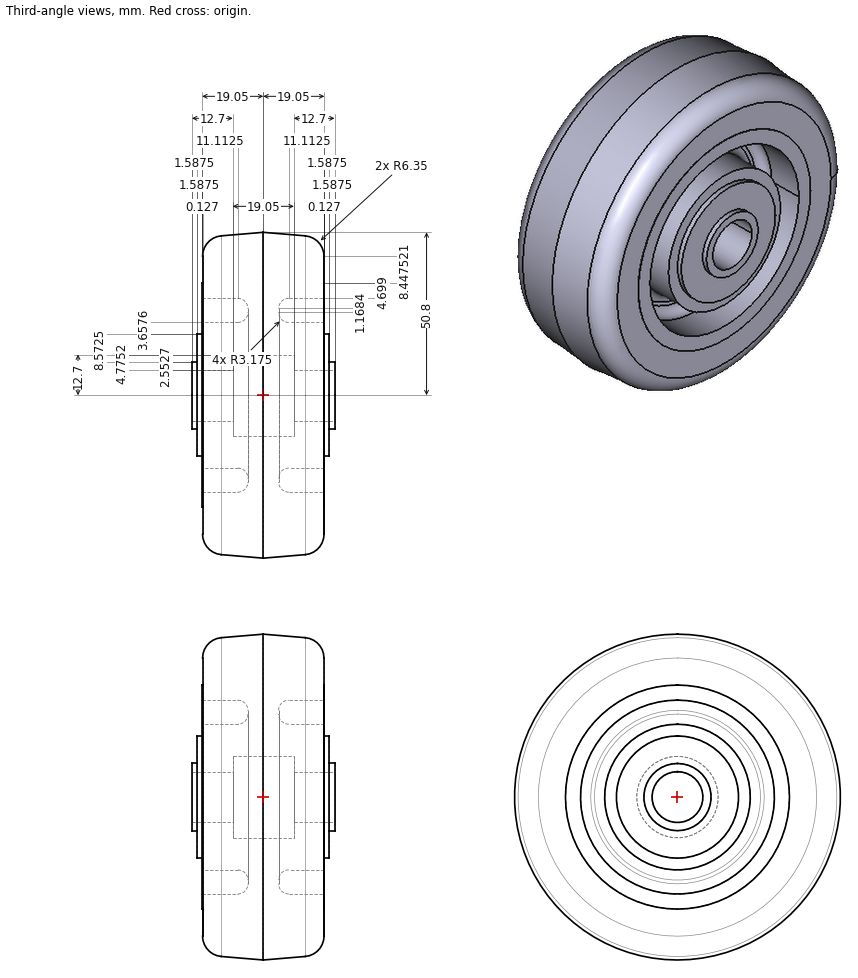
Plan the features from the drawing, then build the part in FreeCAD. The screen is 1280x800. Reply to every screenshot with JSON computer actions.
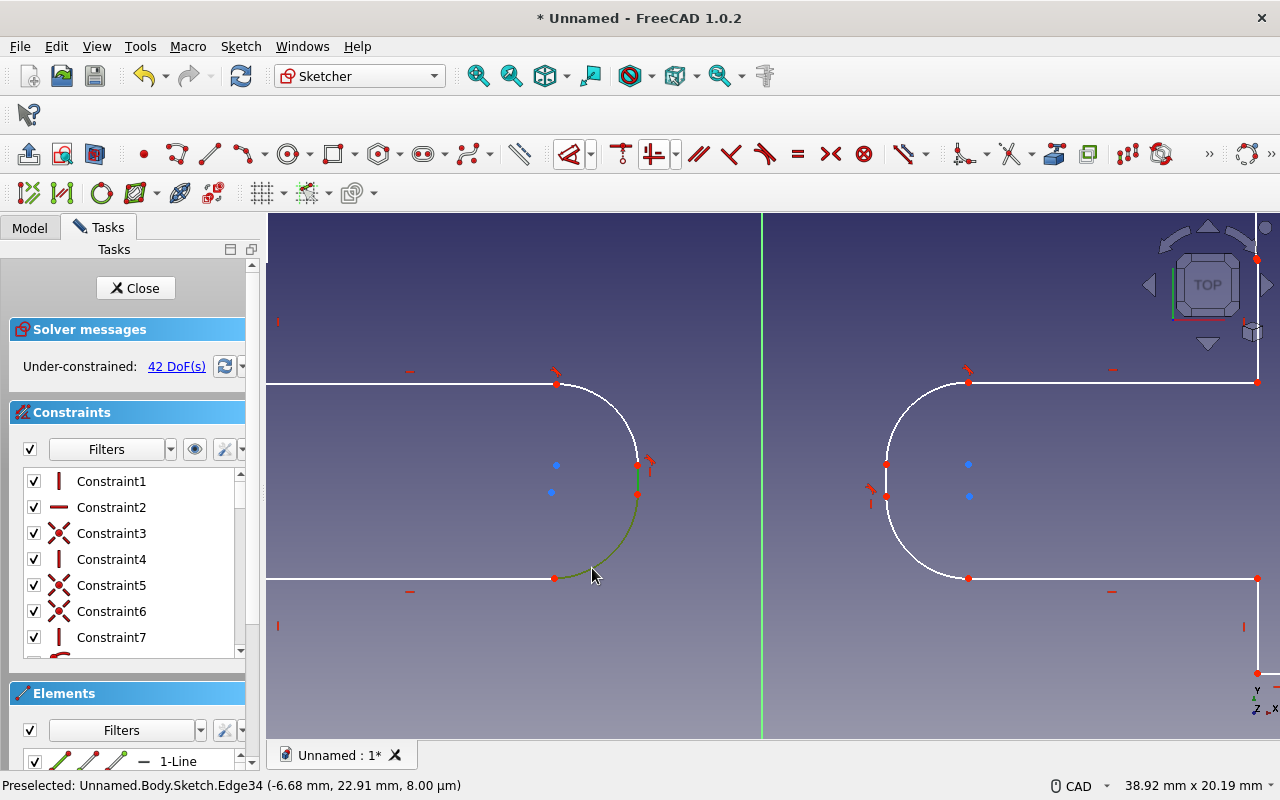
{"action": "left_click", "coordinate": [765, 154]}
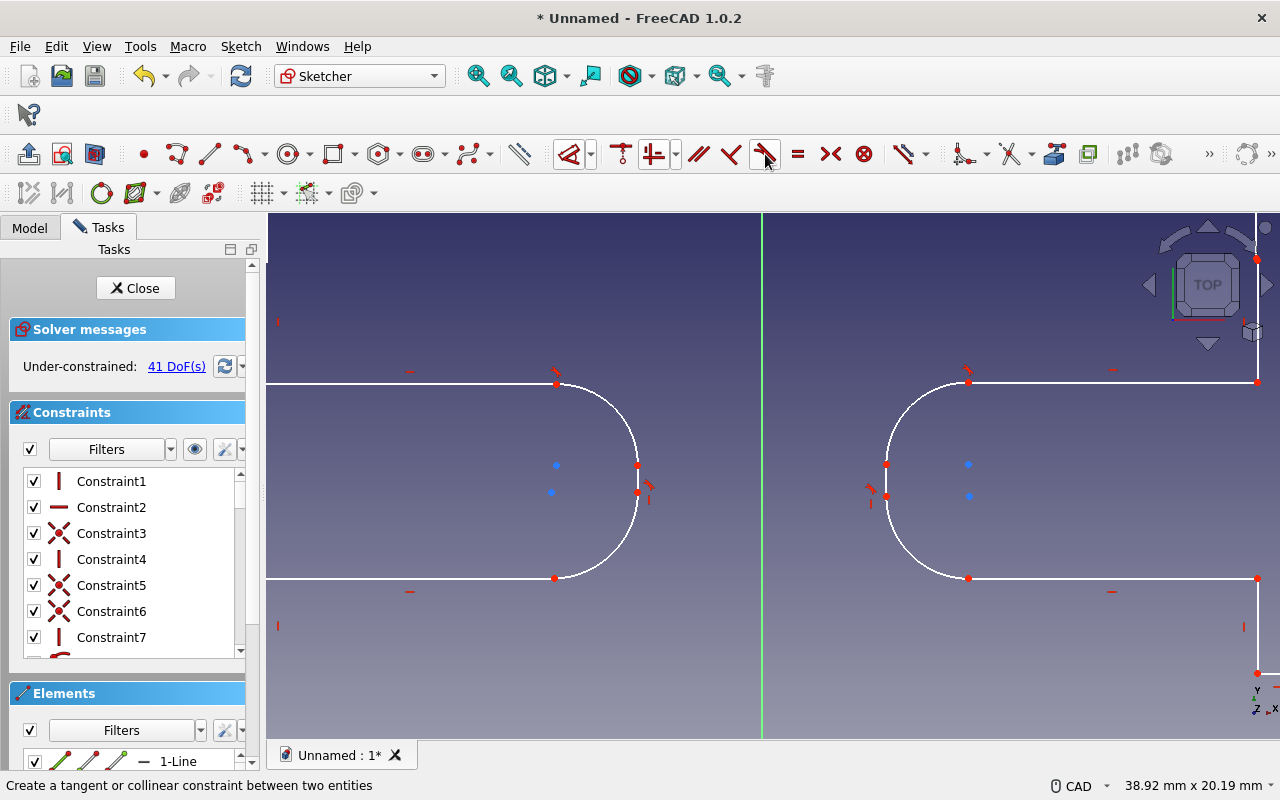
{"action": "scroll", "coordinate": [686, 466], "scroll_direction": "down", "scroll_amount": 7}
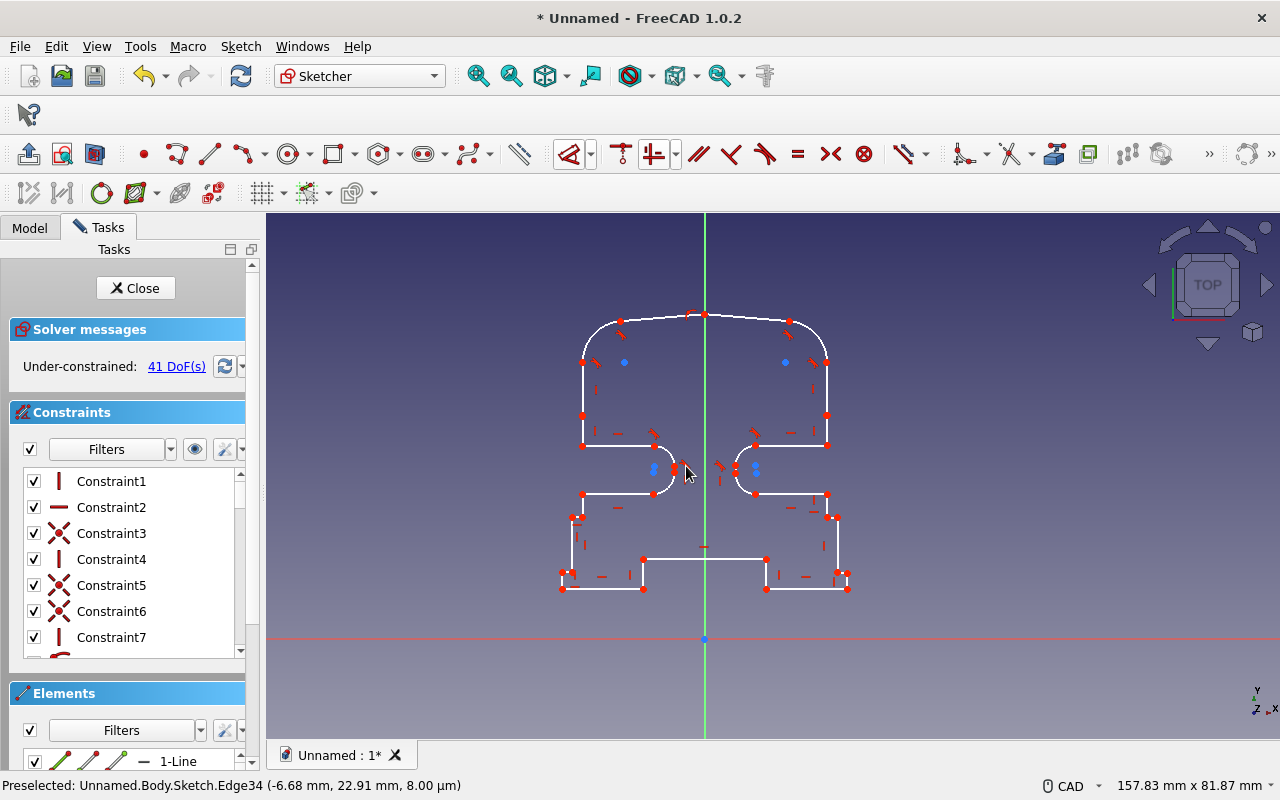
{"action": "left_click", "coordinate": [633, 494]}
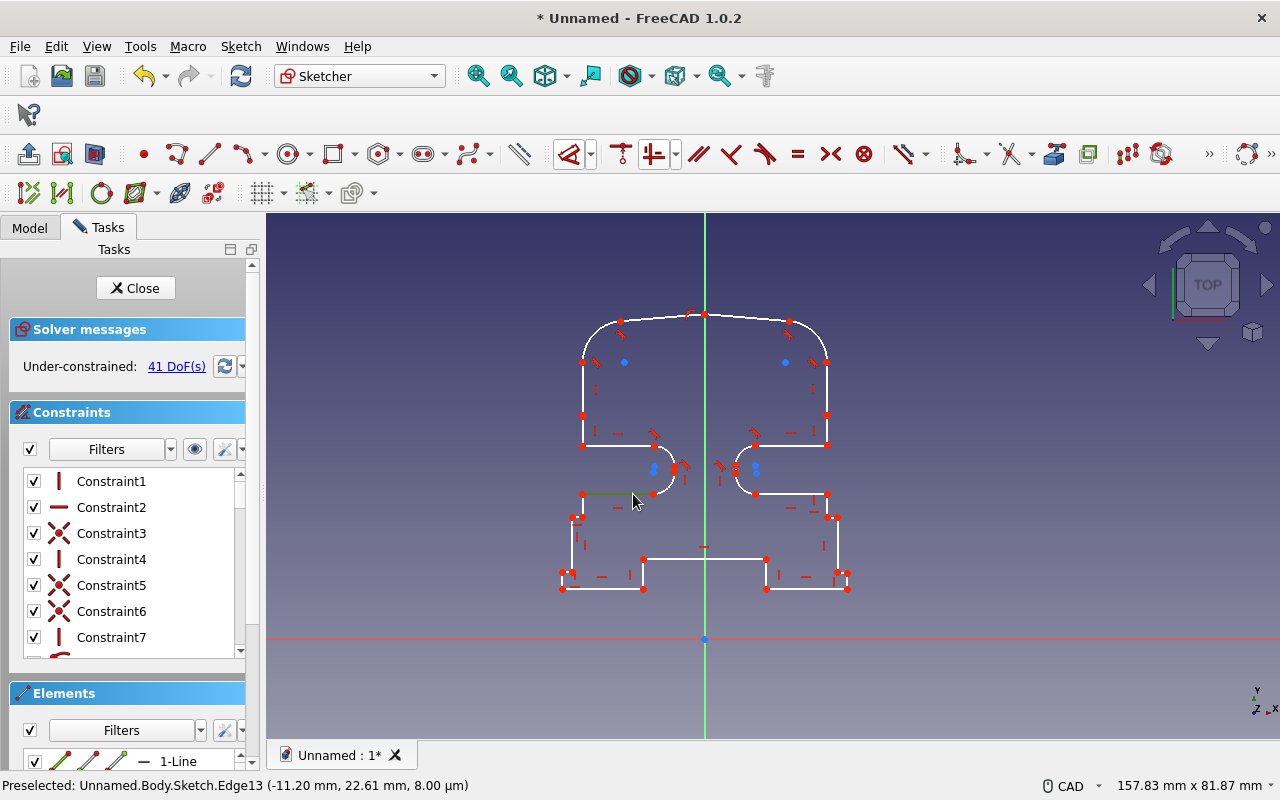
{"action": "scroll", "coordinate": [663, 492], "scroll_direction": "up", "scroll_amount": 2}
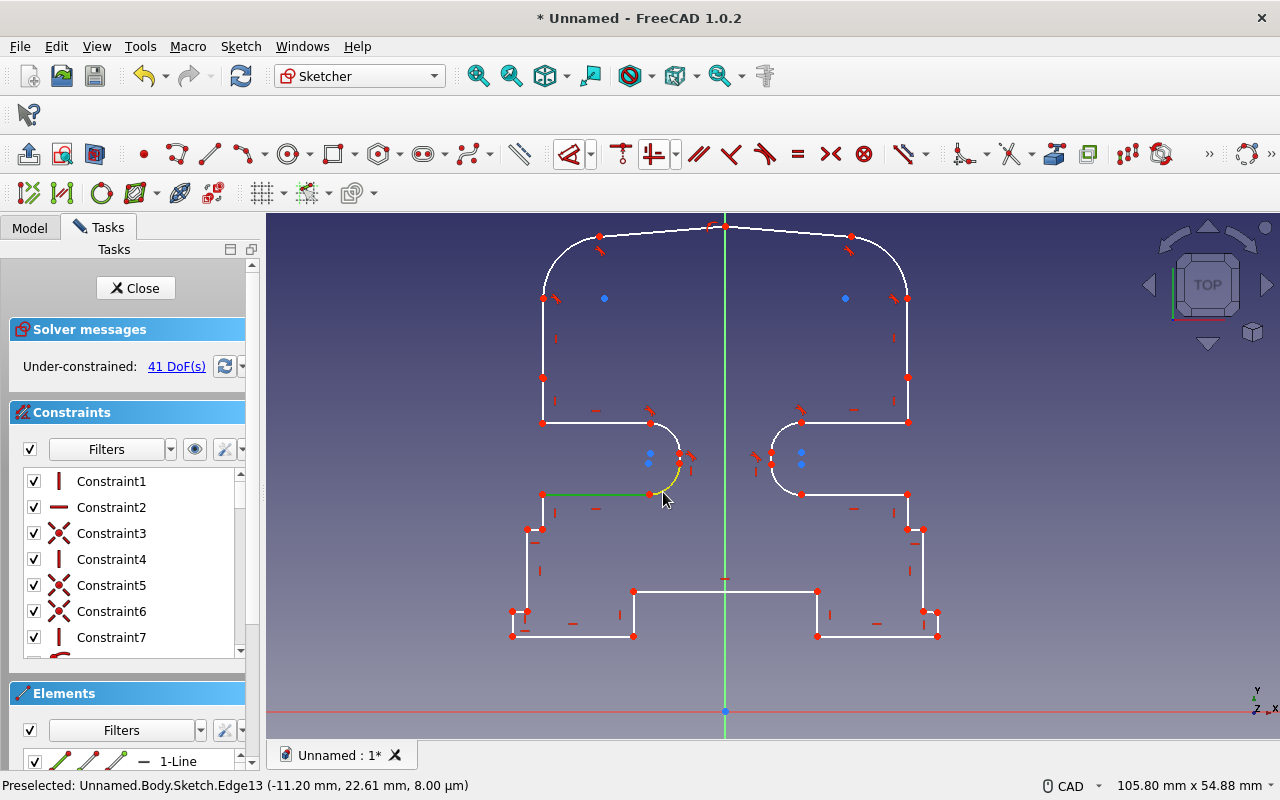
{"action": "left_click", "coordinate": [663, 491]}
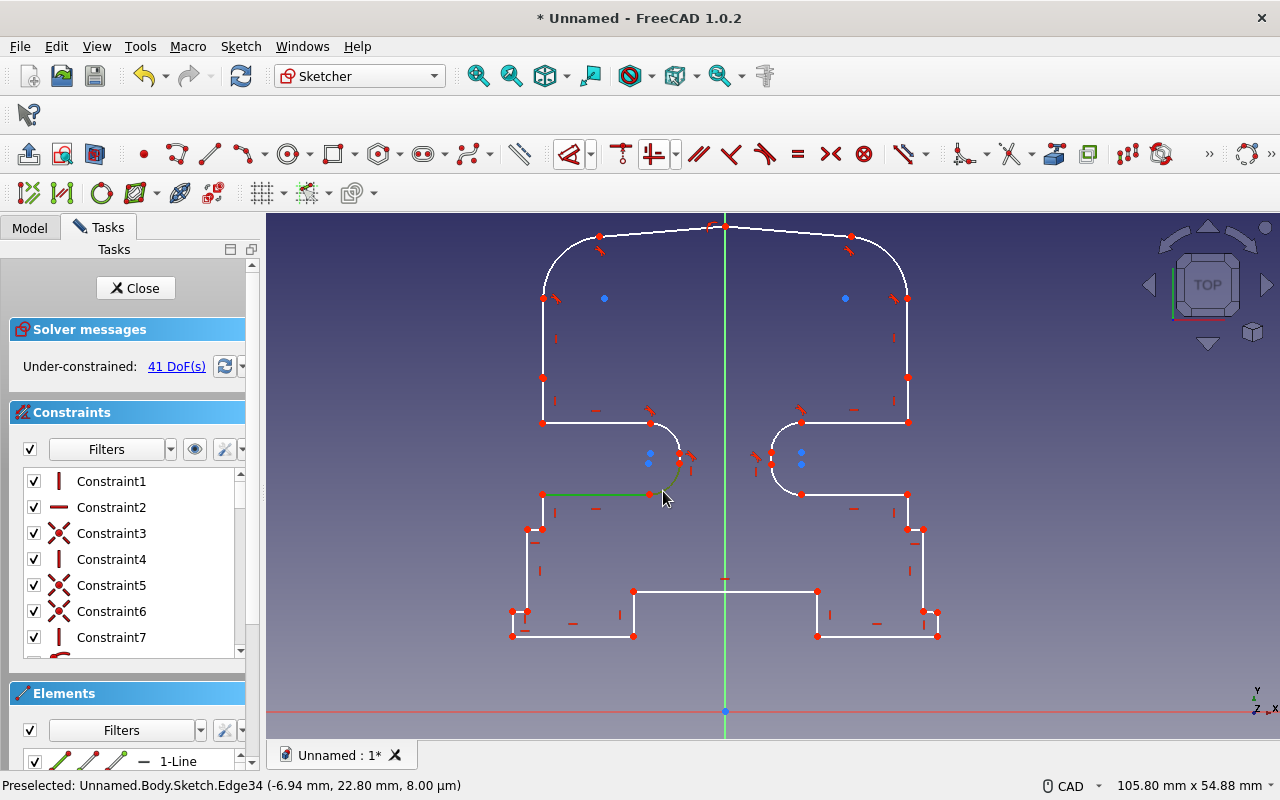
{"action": "left_click", "coordinate": [765, 154]}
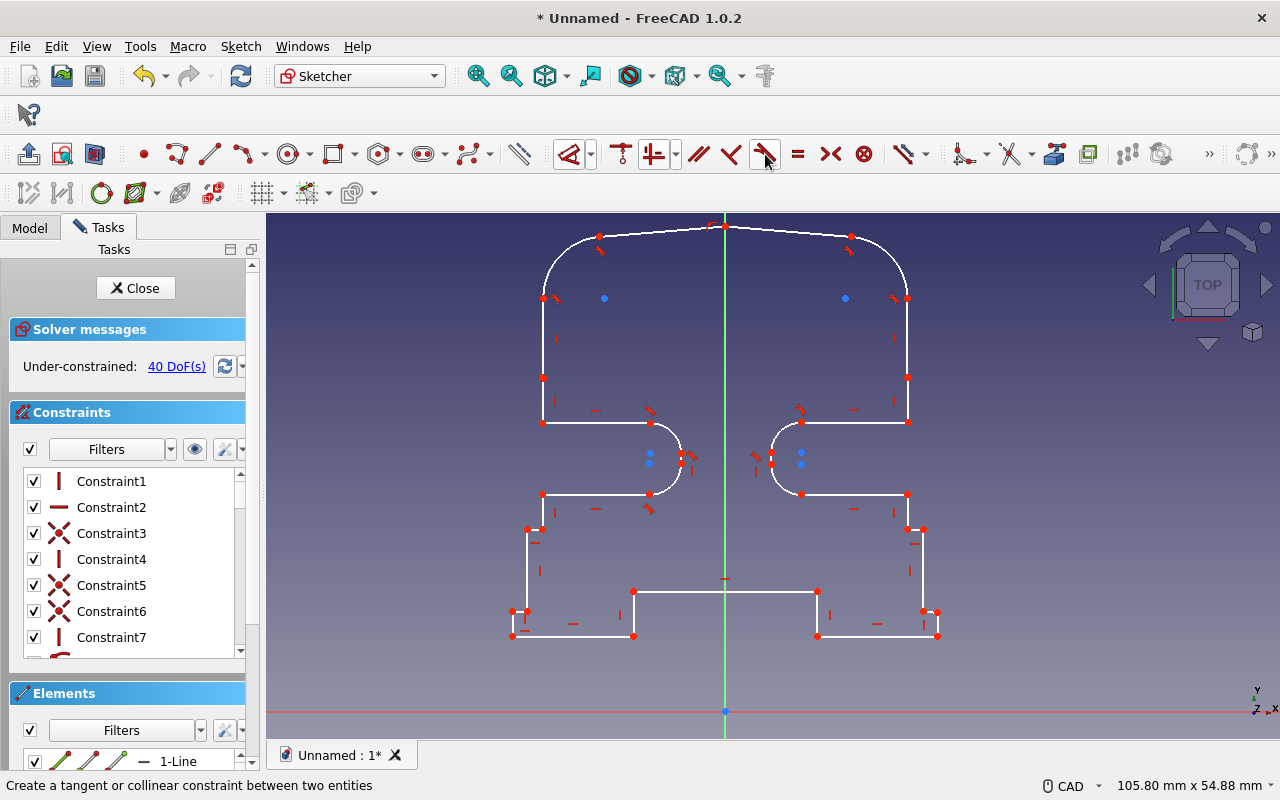
{"action": "left_click", "coordinate": [876, 495]}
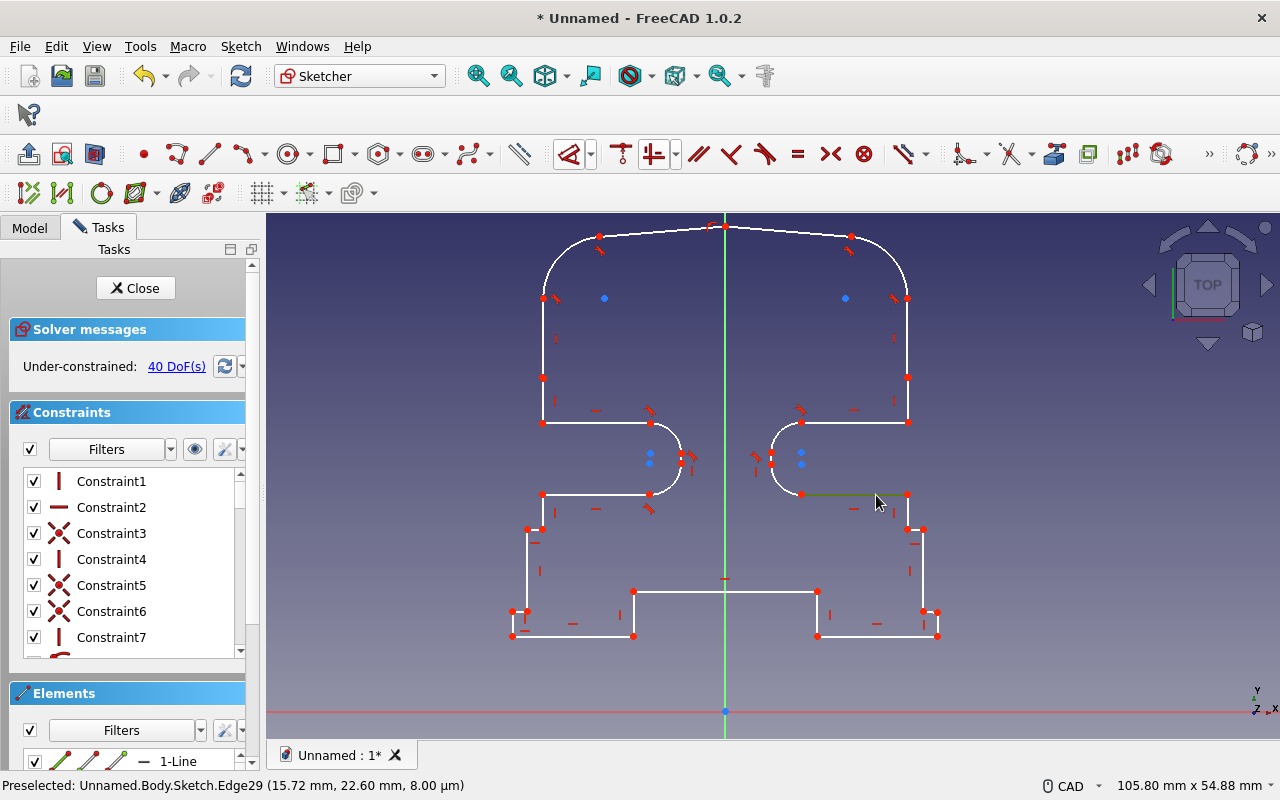
{"action": "left_click", "coordinate": [775, 478]}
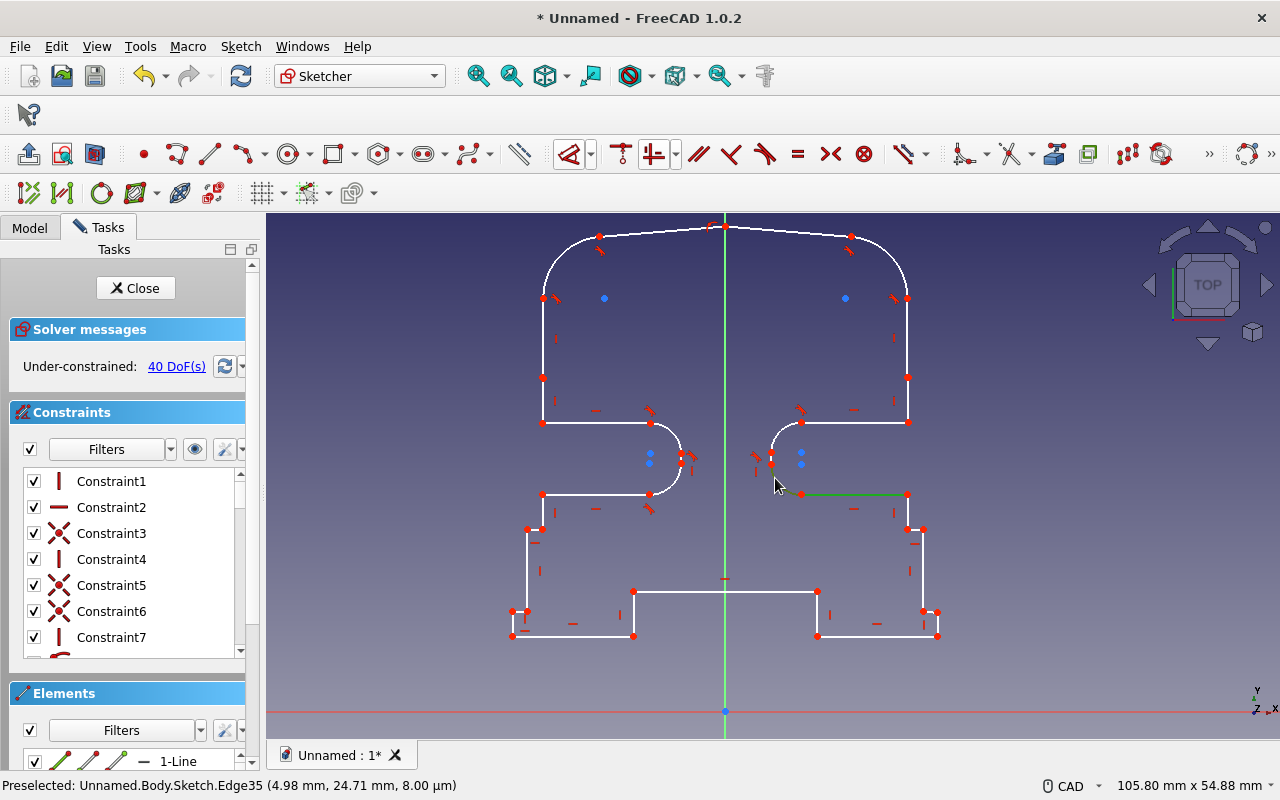
{"action": "left_click", "coordinate": [765, 154]}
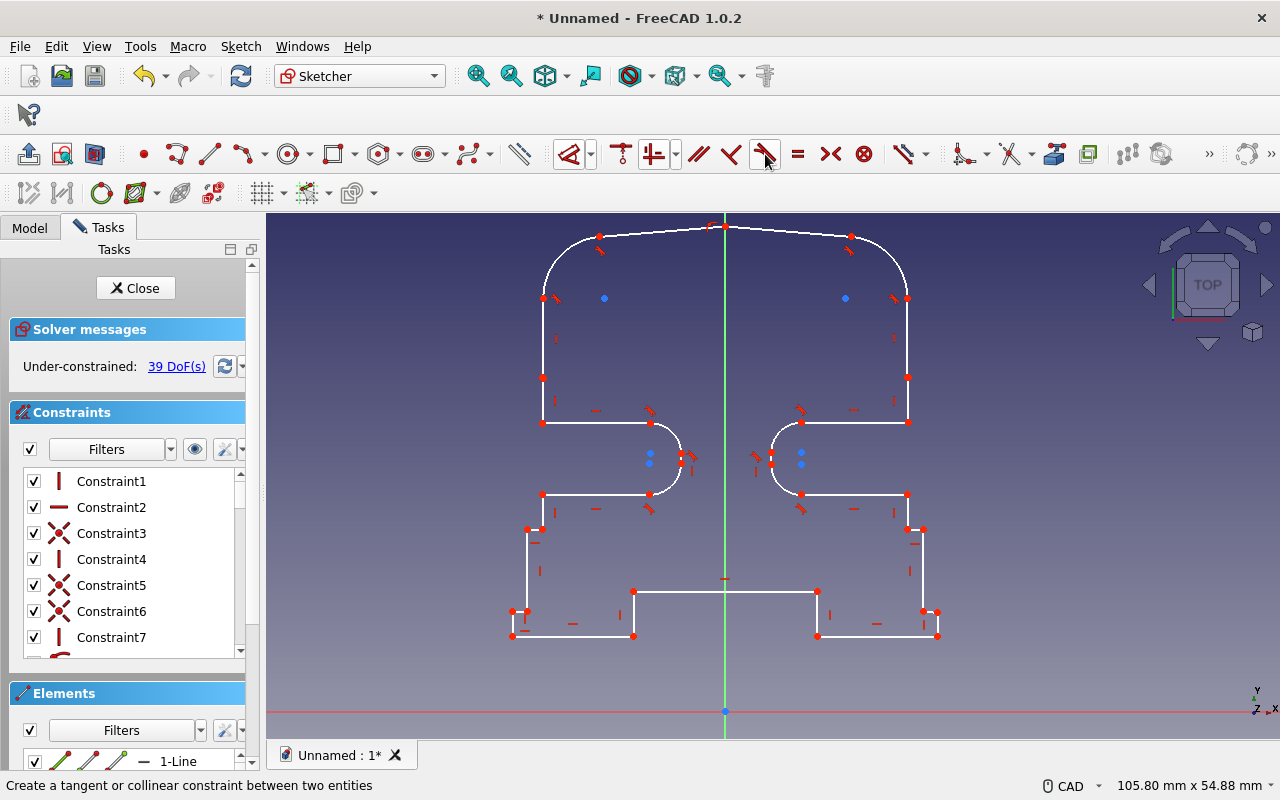
{"action": "scroll", "coordinate": [908, 378], "scroll_direction": "up", "scroll_amount": 12}